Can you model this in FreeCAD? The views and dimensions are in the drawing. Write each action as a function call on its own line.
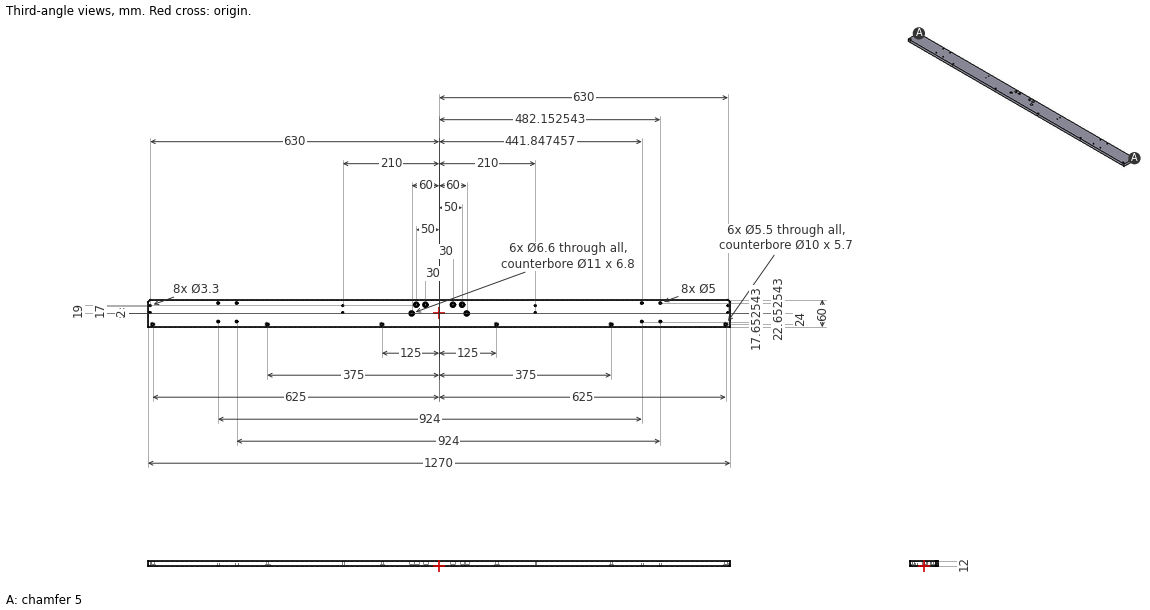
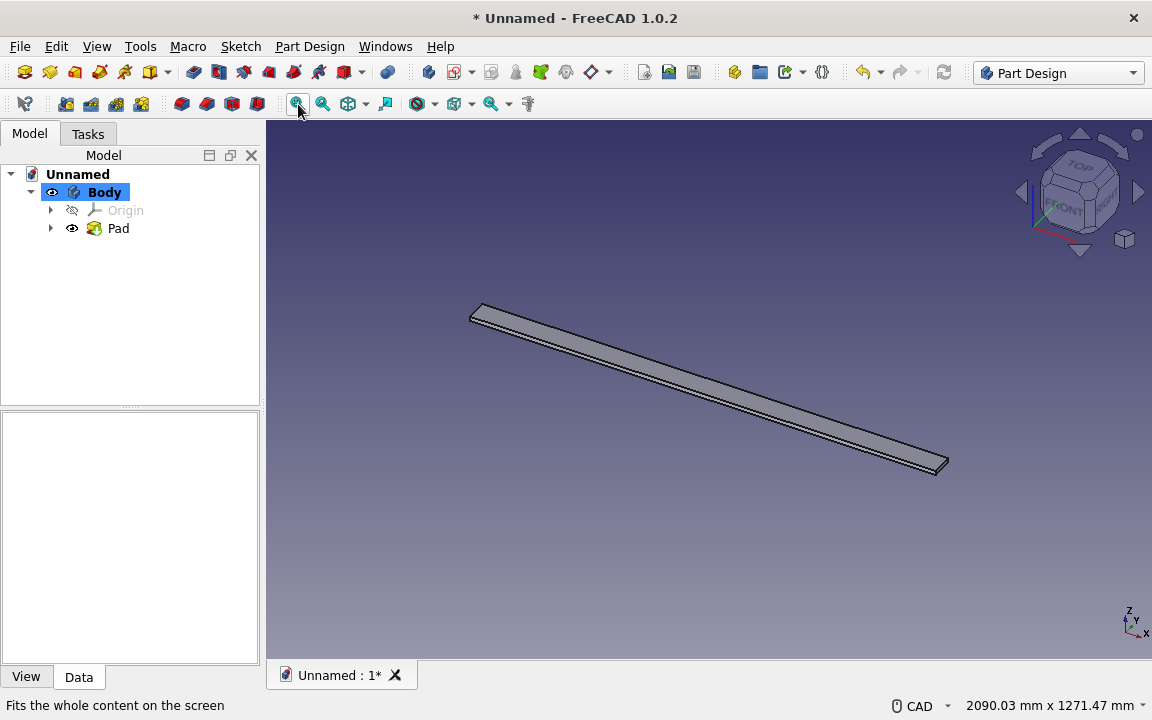
scroll(482, 305, up, 11)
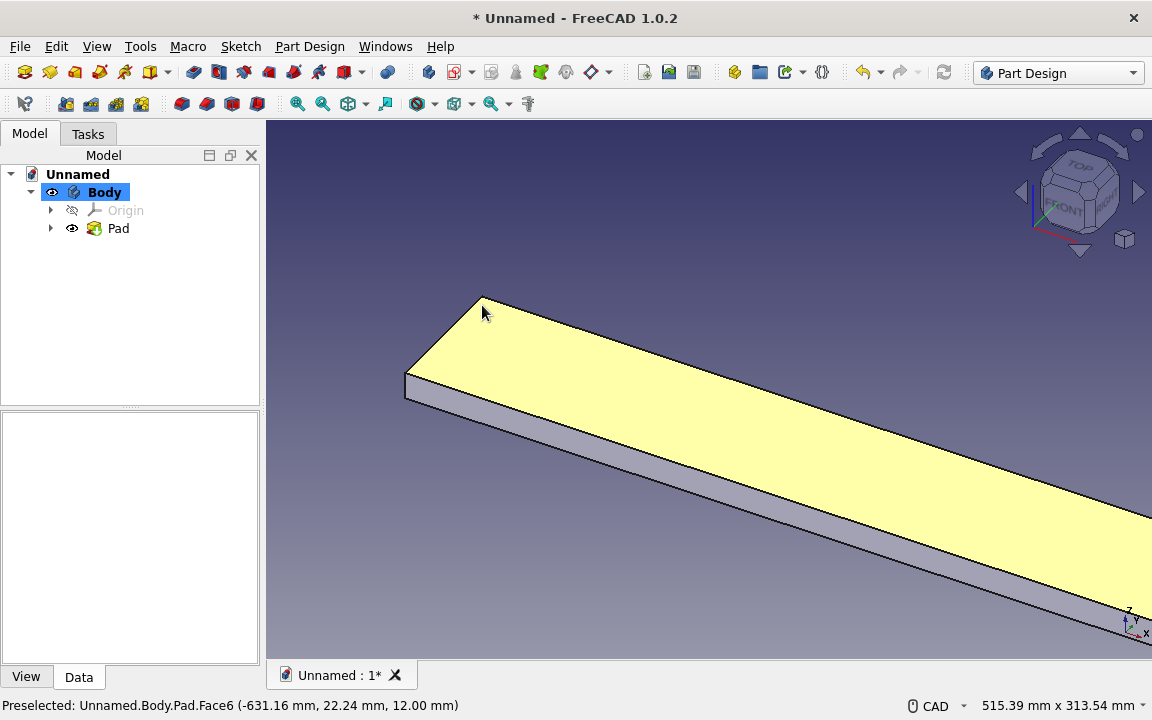
click(298, 104)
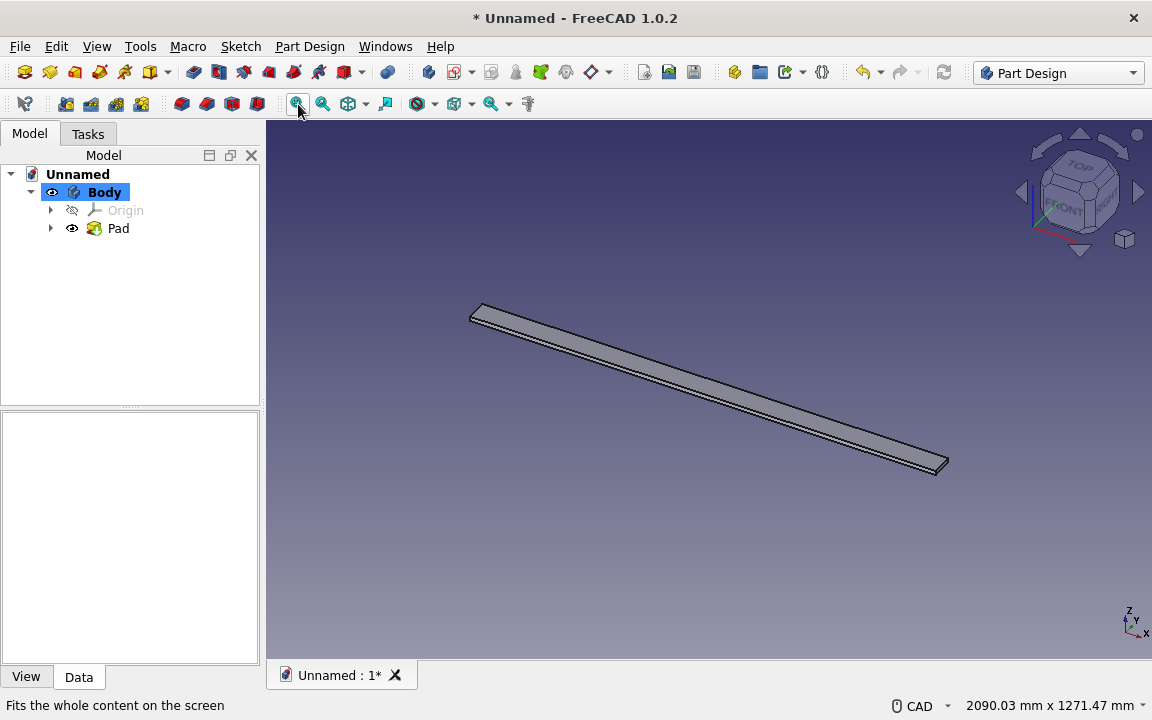
key(0)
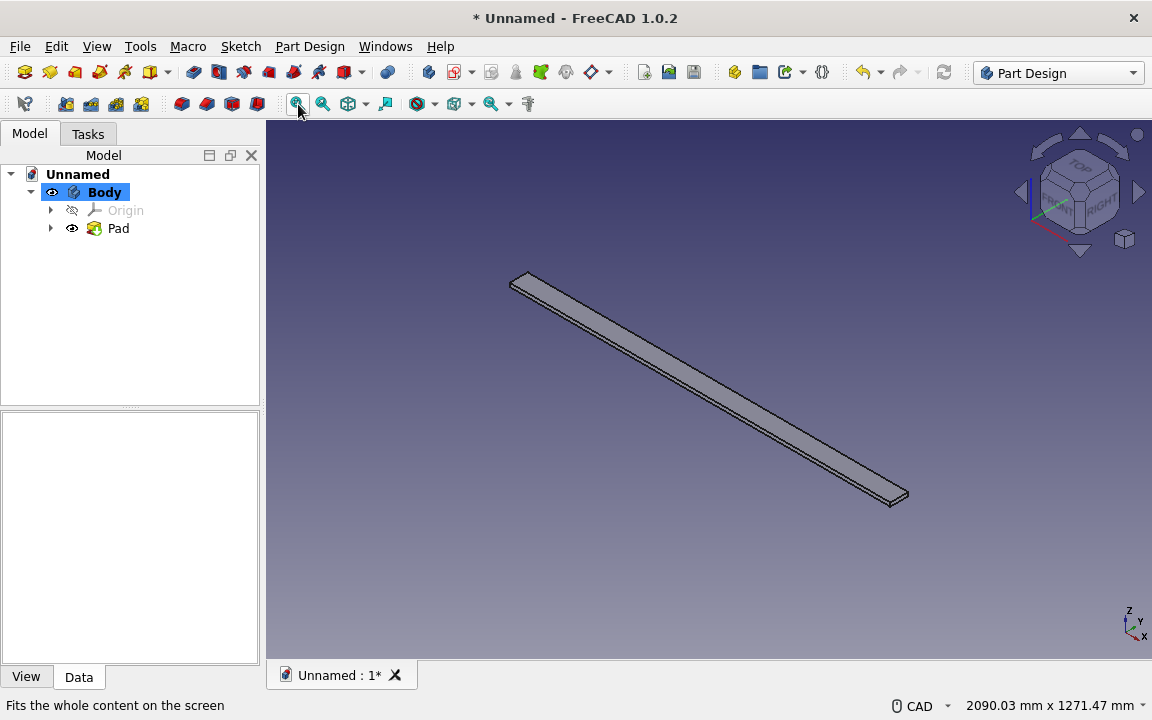
click(298, 104)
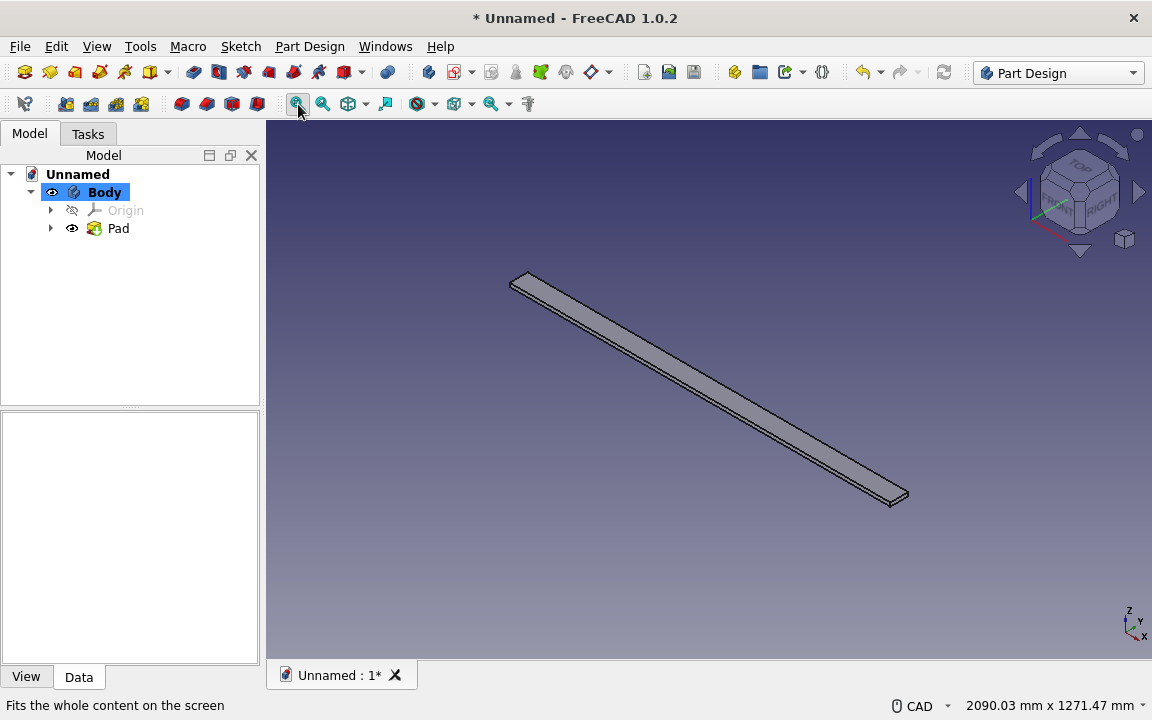
scroll(528, 273, up, 11)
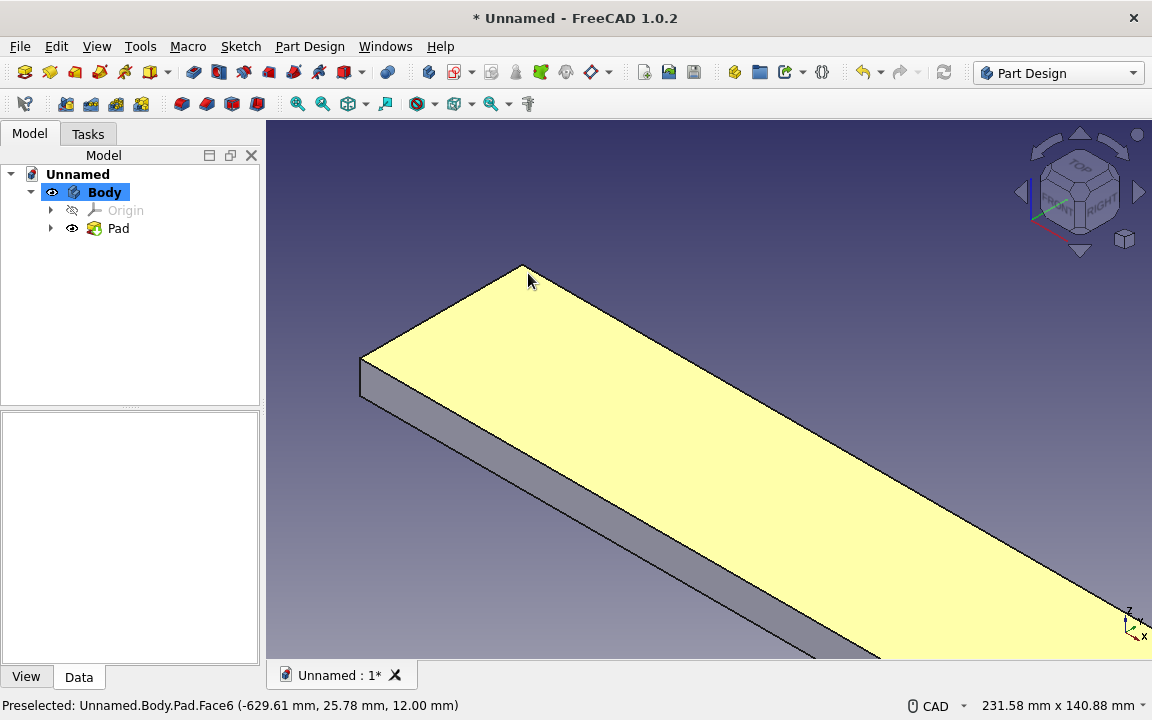
key(v)
key(f)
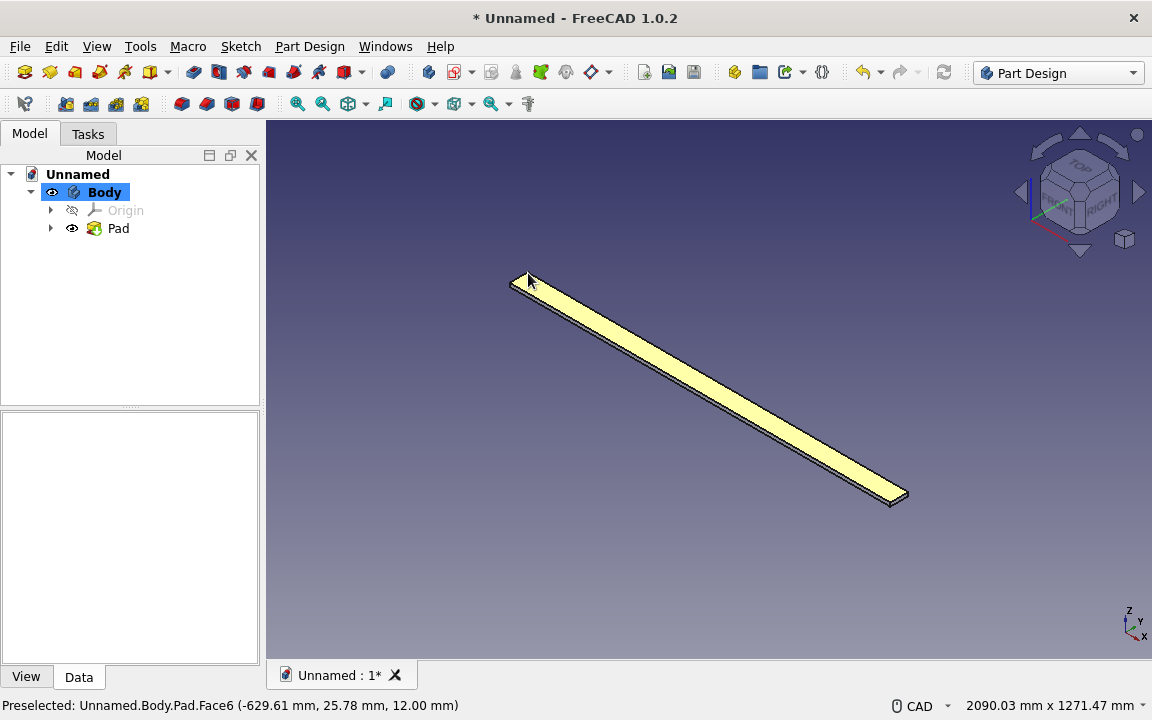
key(2)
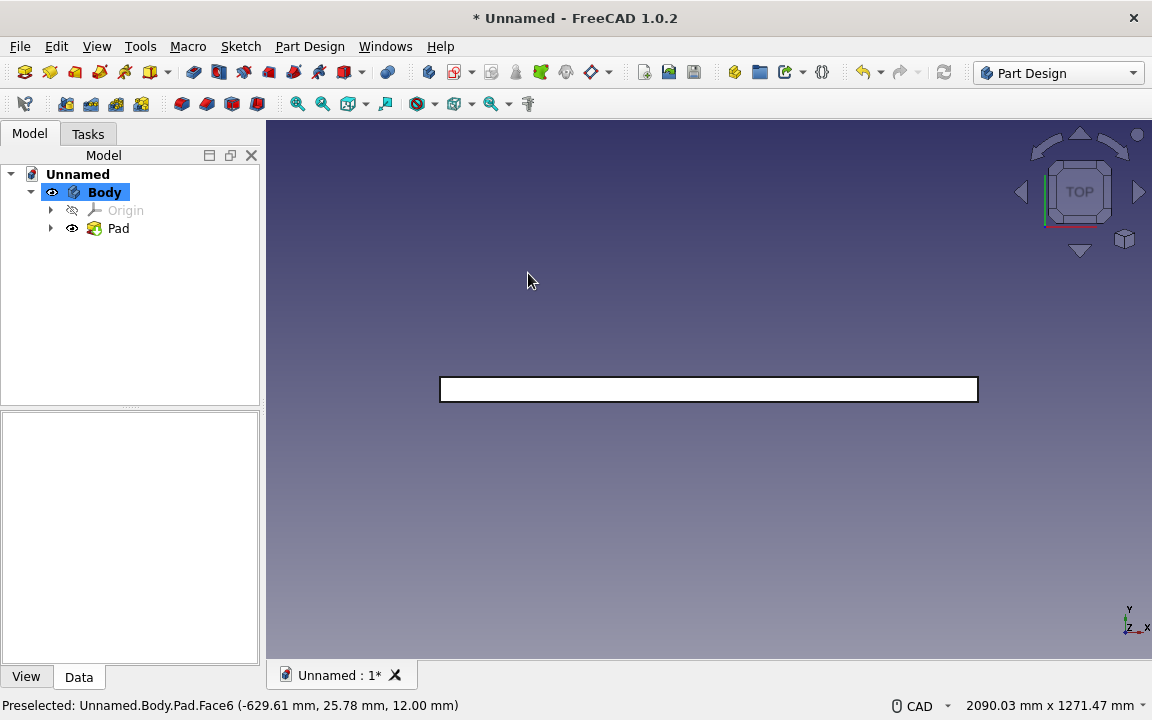
scroll(440, 376, up, 11)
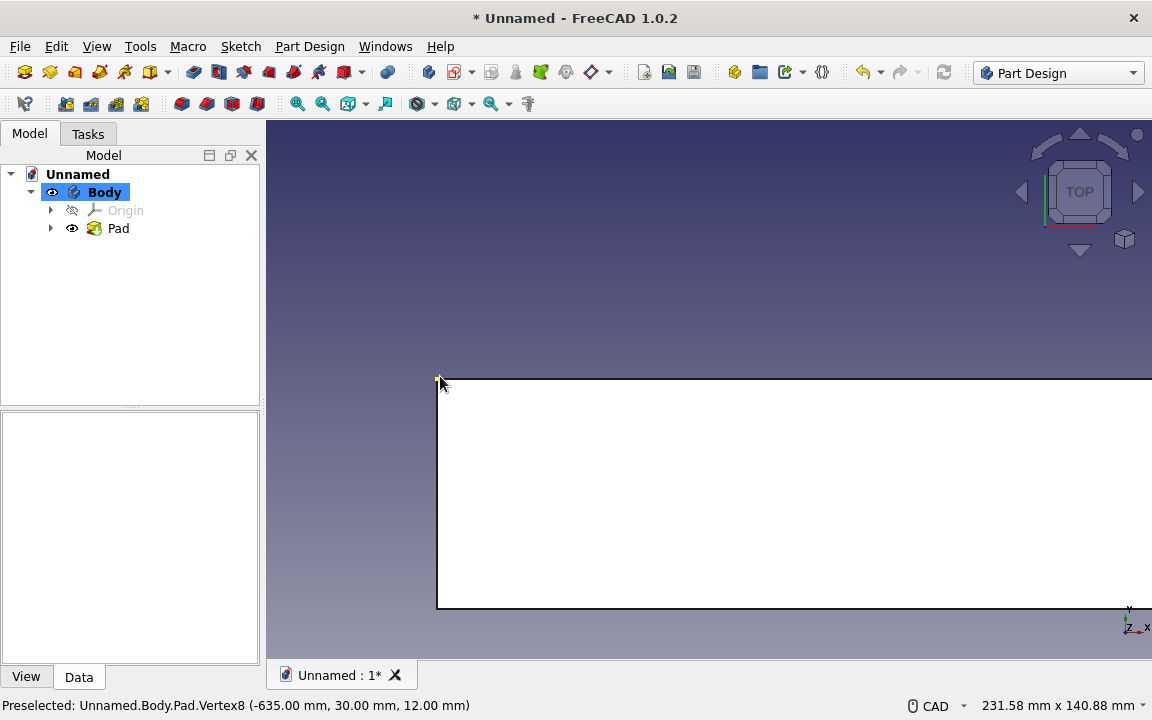
click(298, 104)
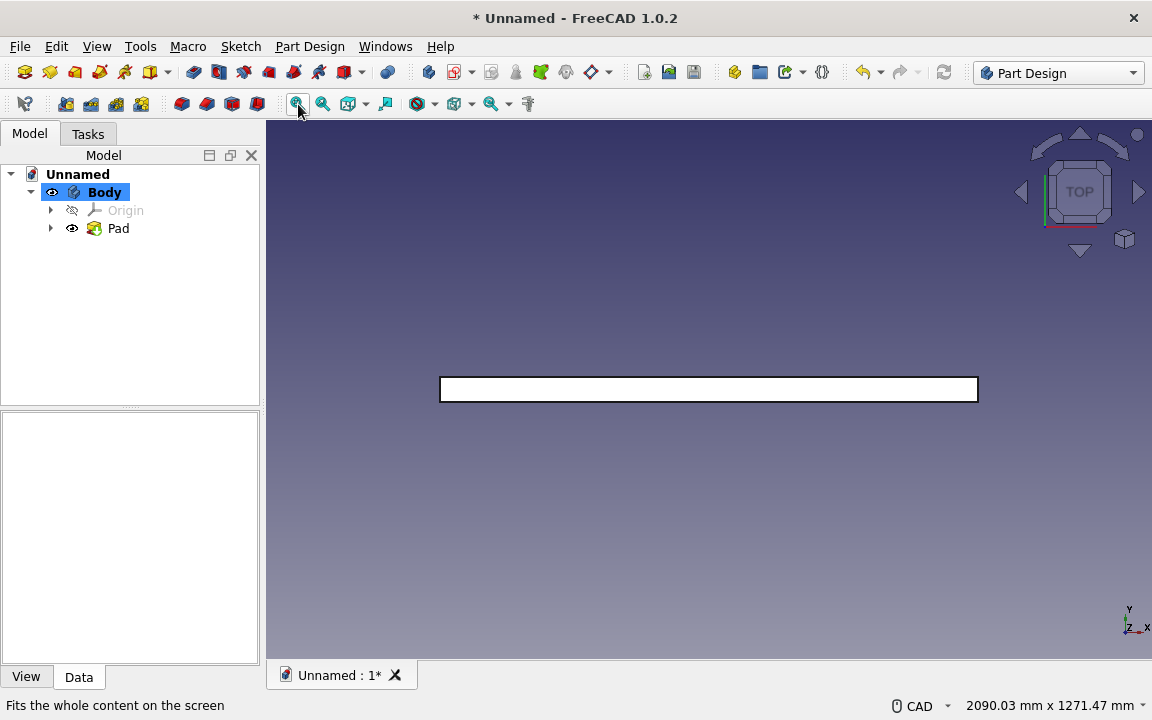
key(1)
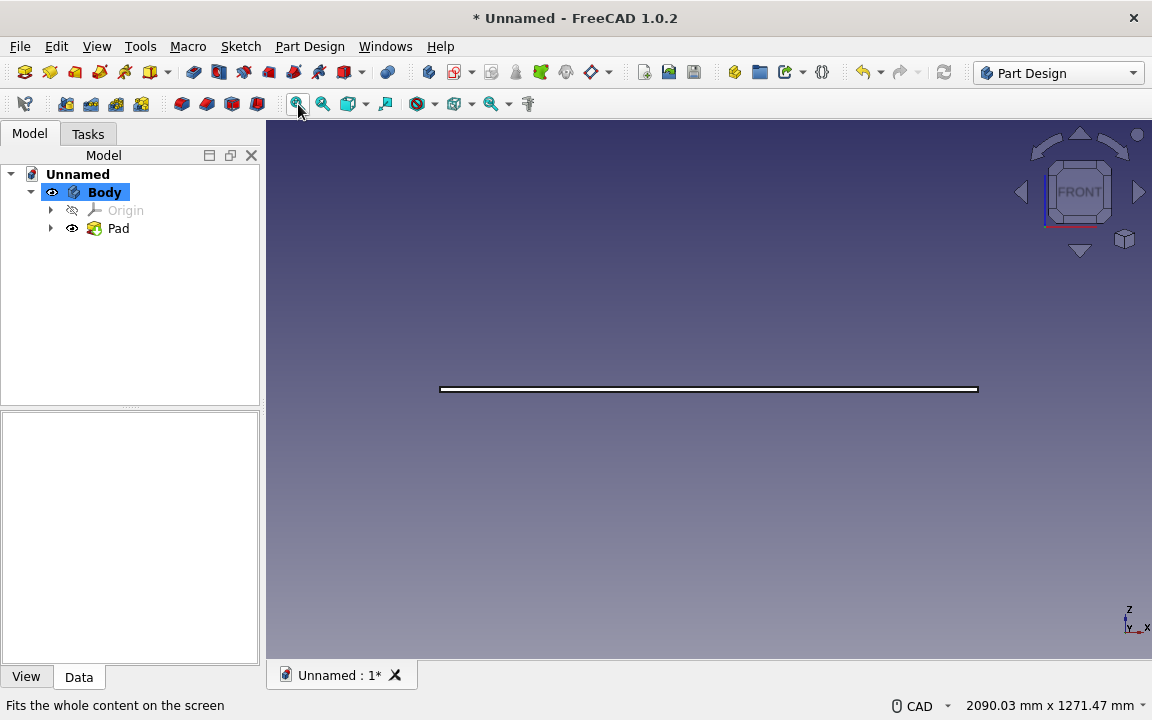
scroll(440, 388, up, 11)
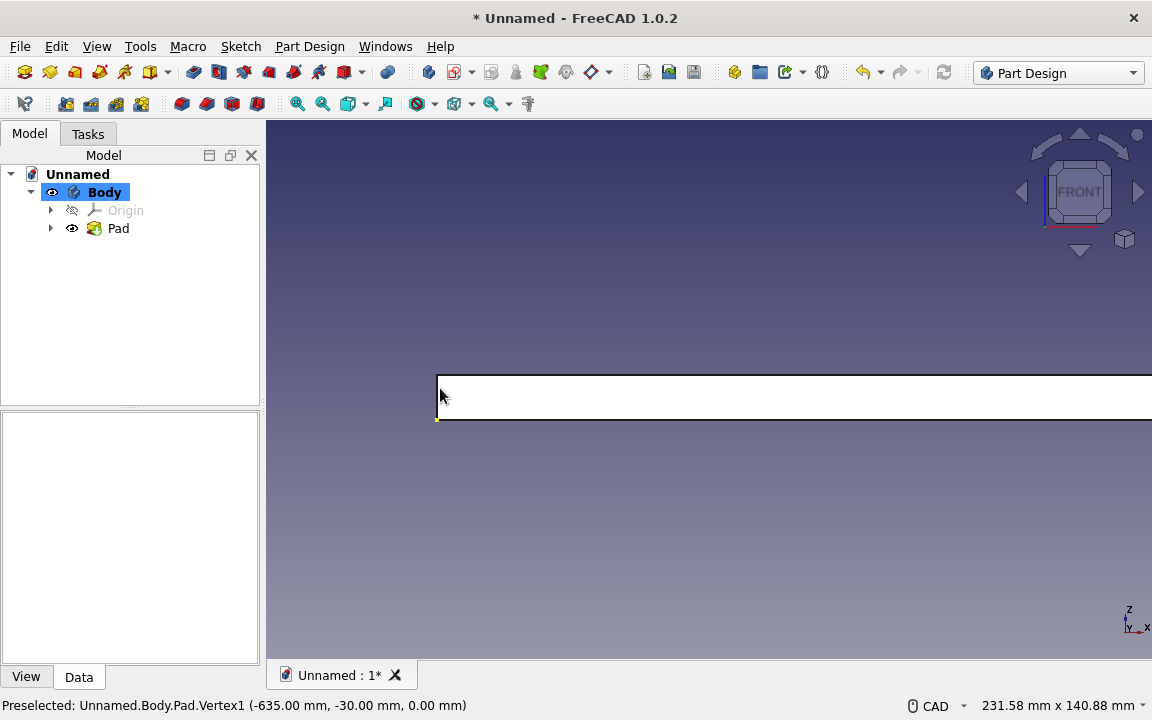
key(v)
key(f)